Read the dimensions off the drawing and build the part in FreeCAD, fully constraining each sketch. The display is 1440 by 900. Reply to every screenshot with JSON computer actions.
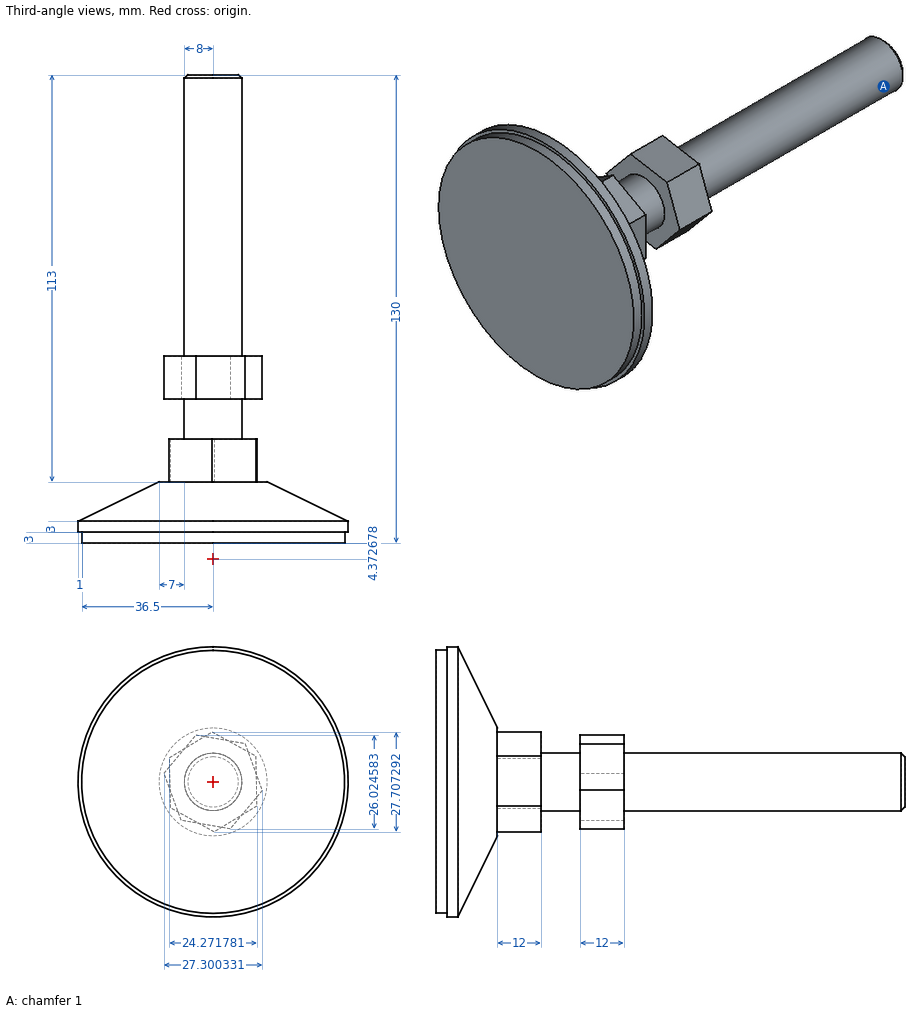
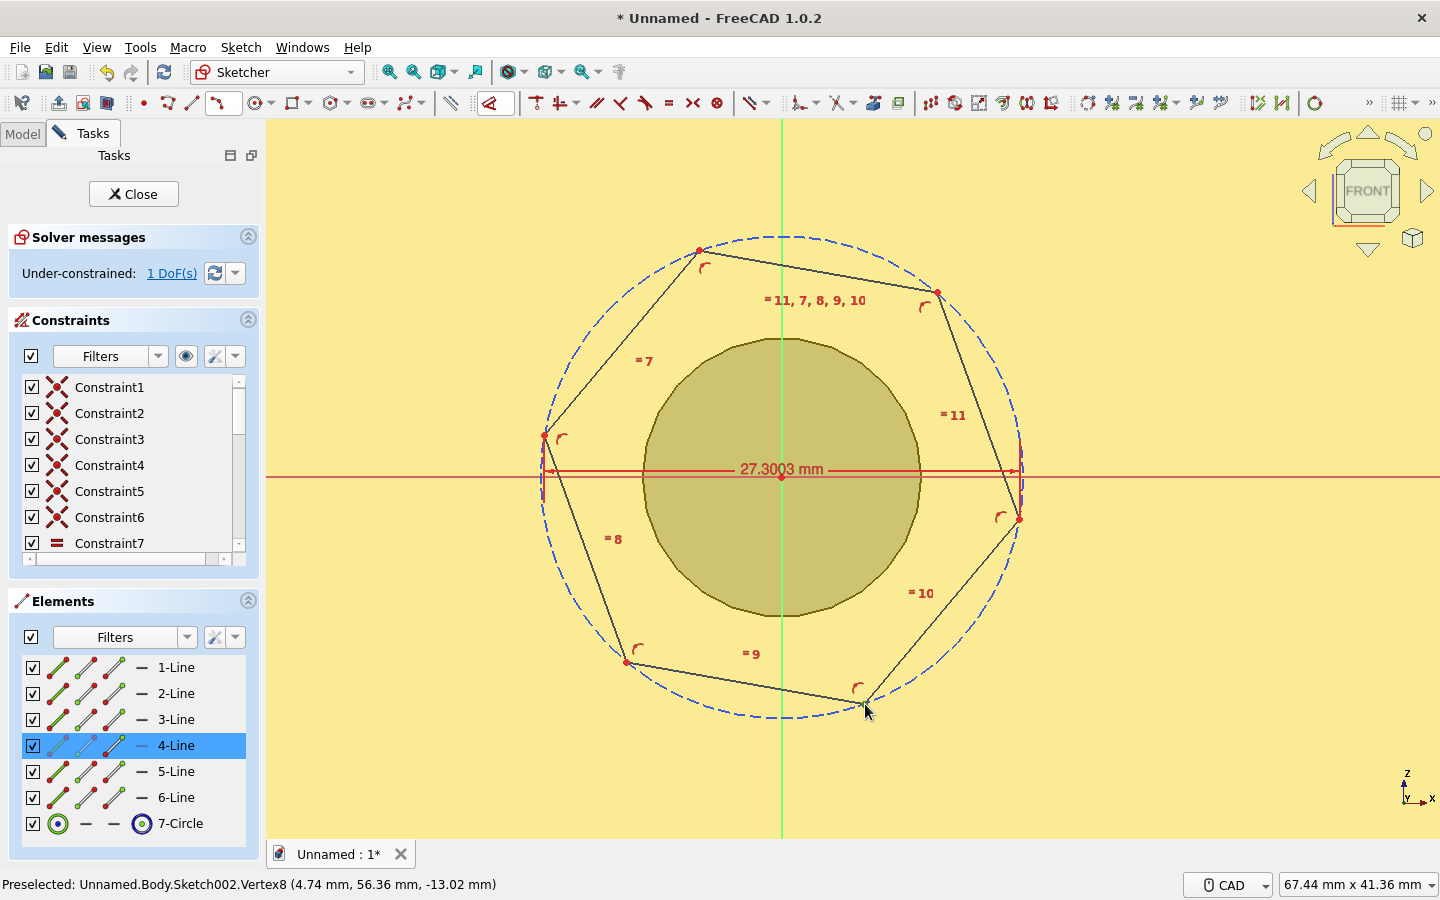
{"action": "left_click", "coordinate": [699, 251]}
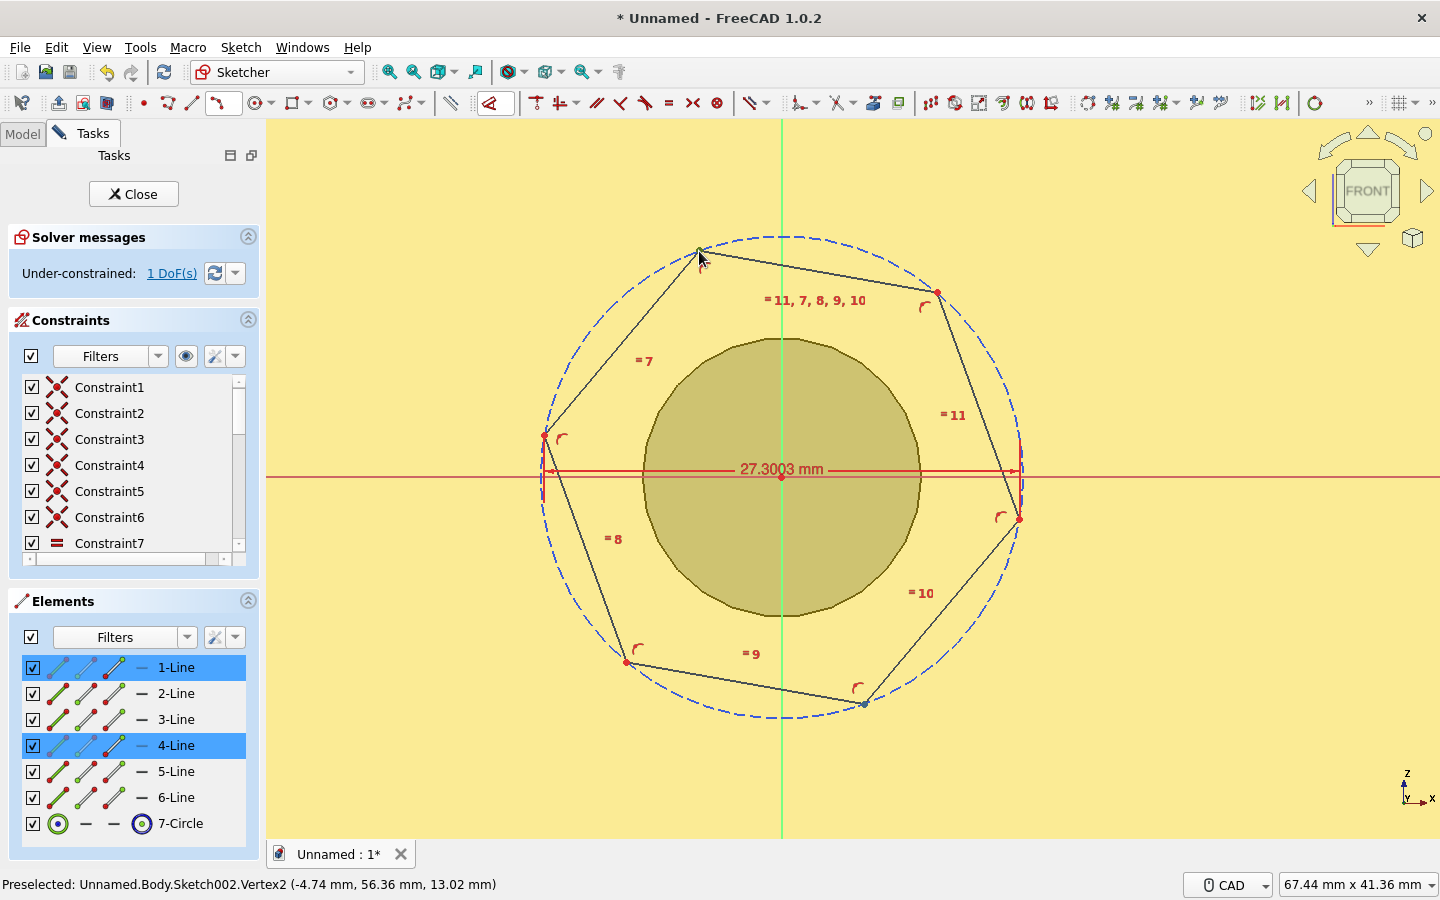
{"action": "left_click", "coordinate": [508, 104]}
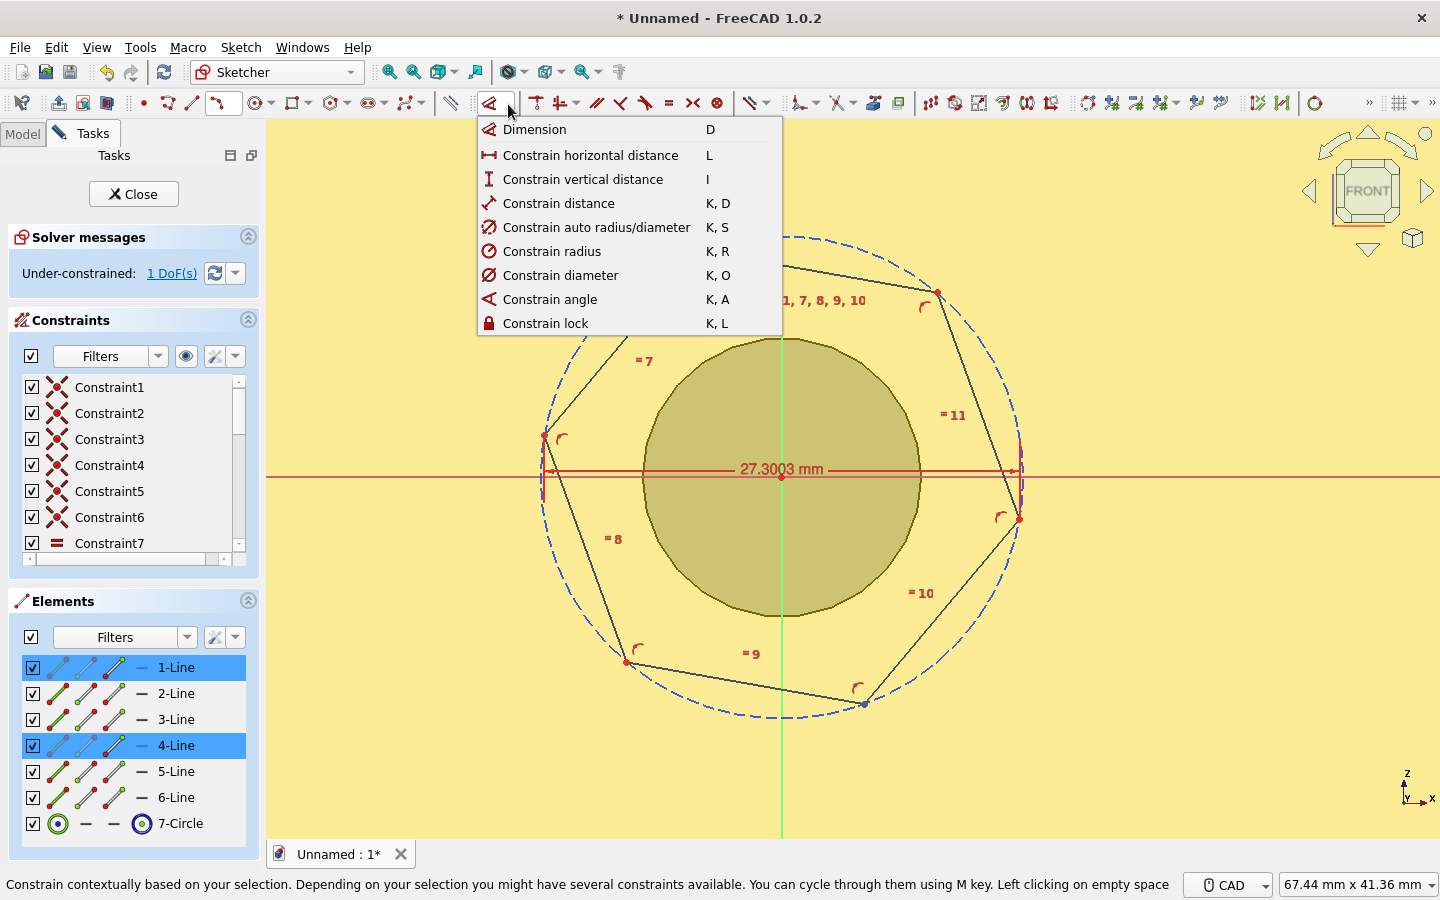
{"action": "left_click", "coordinate": [630, 179]}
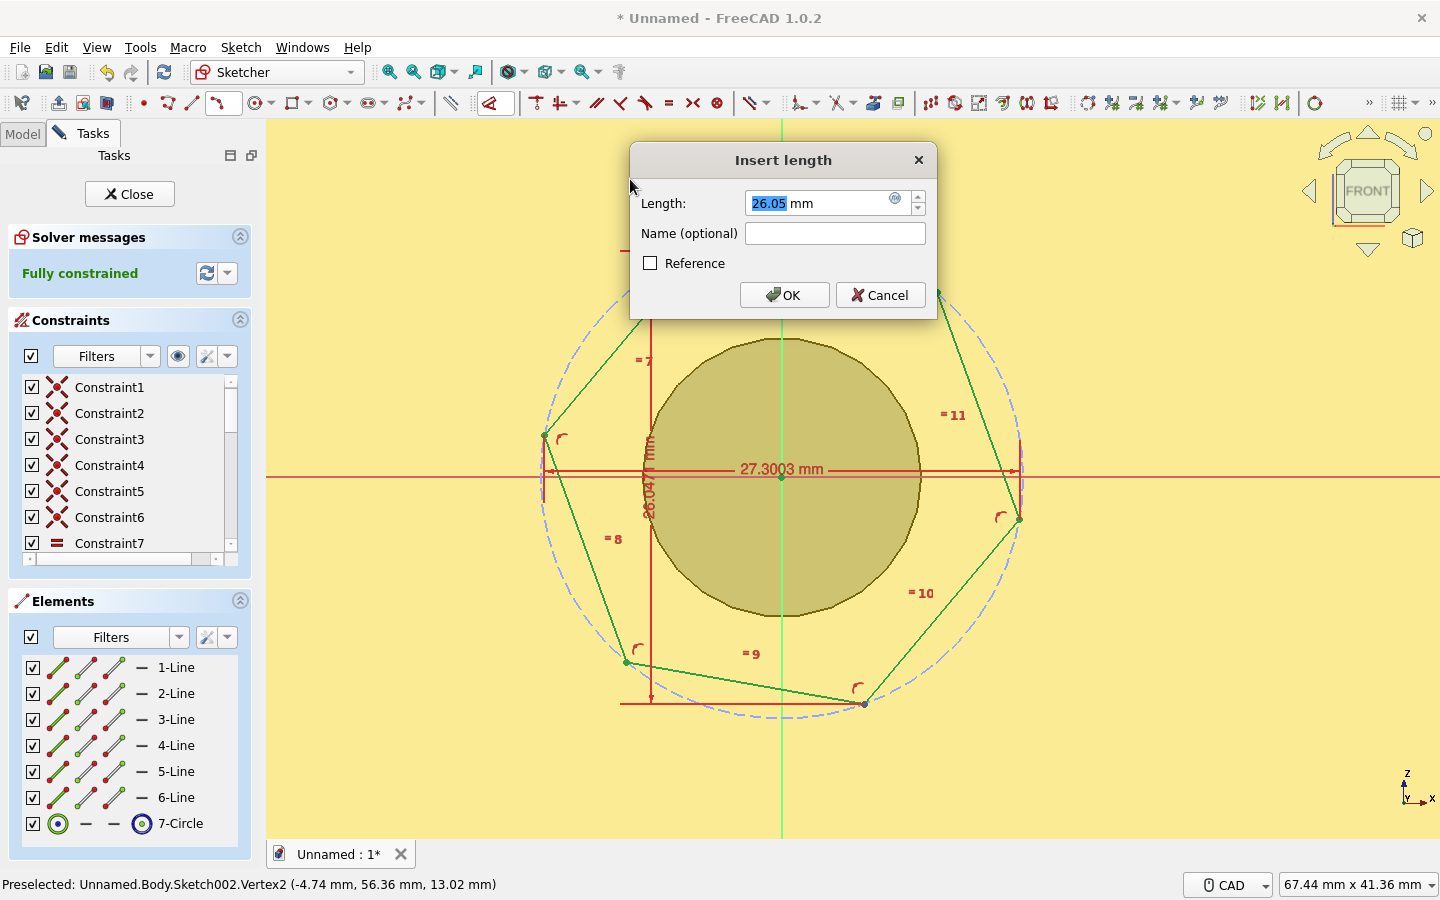
{"action": "type", "text": "26.024583"}
{"action": "key", "text": "Return"}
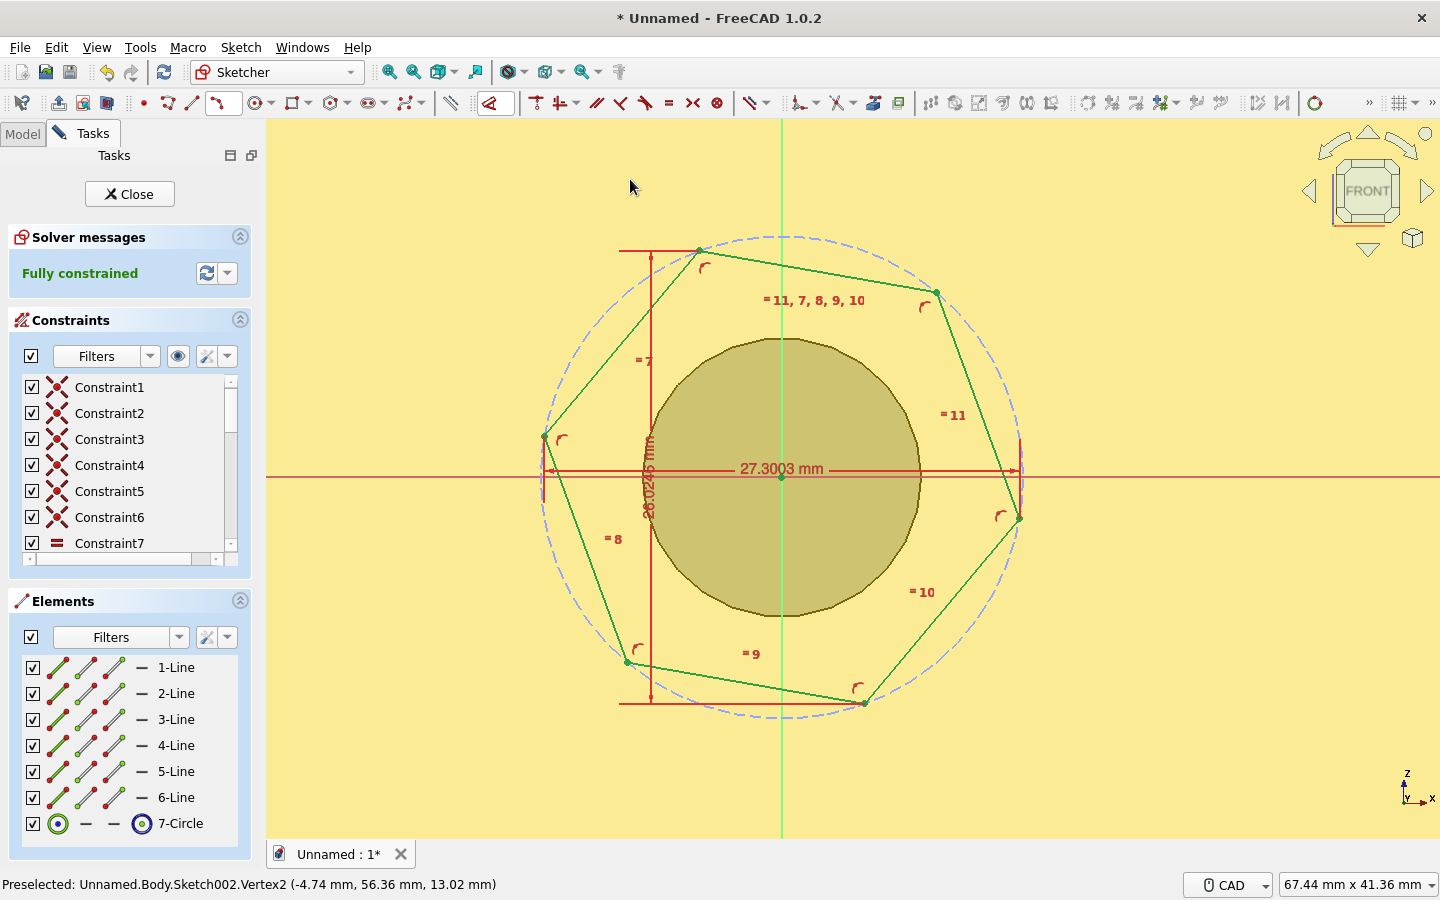
{"action": "left_click", "coordinate": [130, 194]}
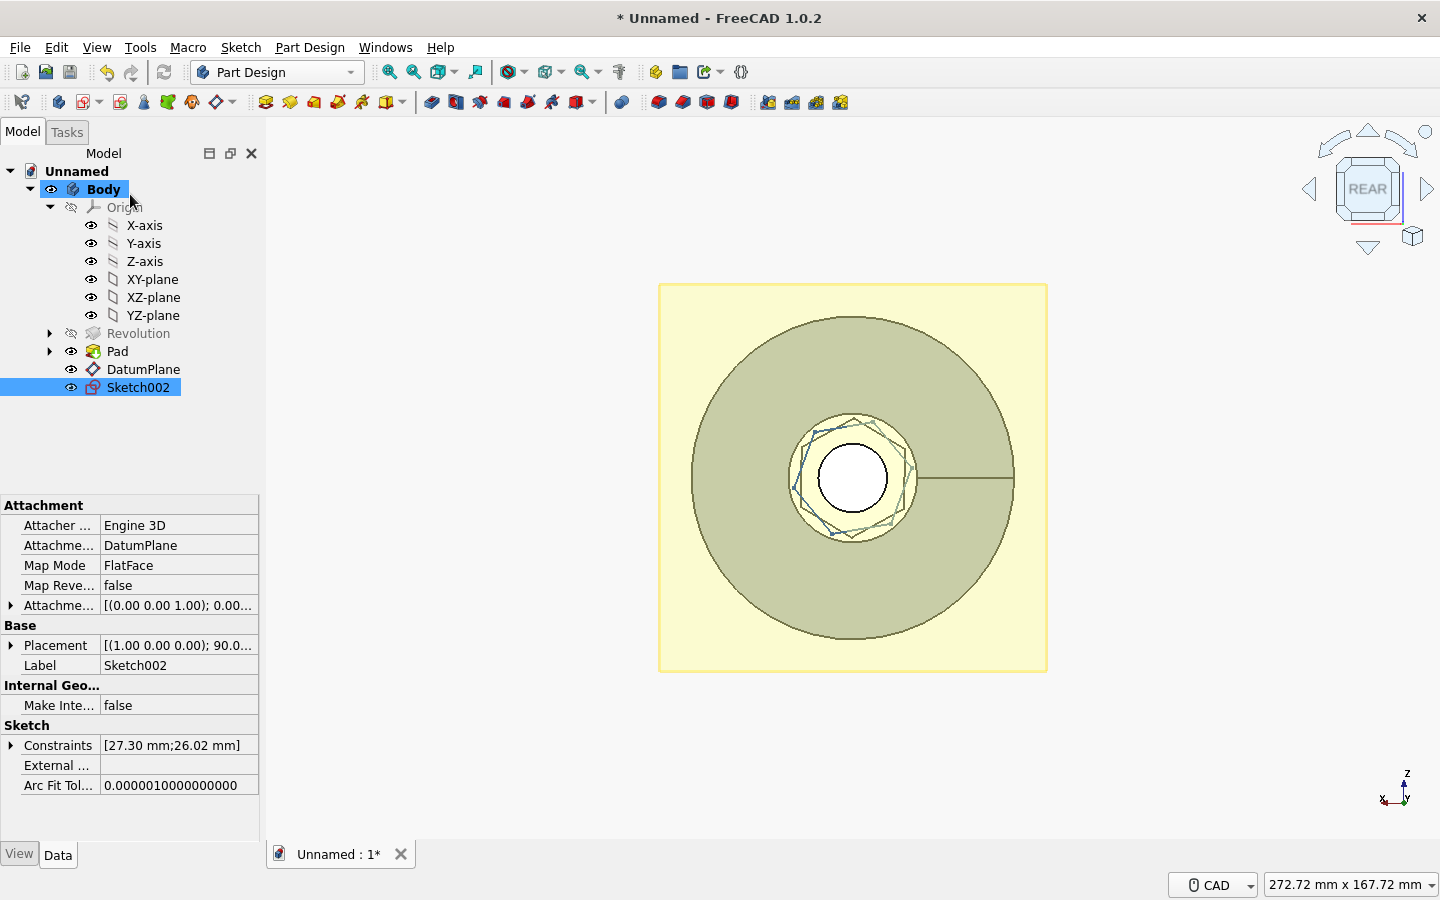
{"action": "left_click", "coordinate": [266, 102]}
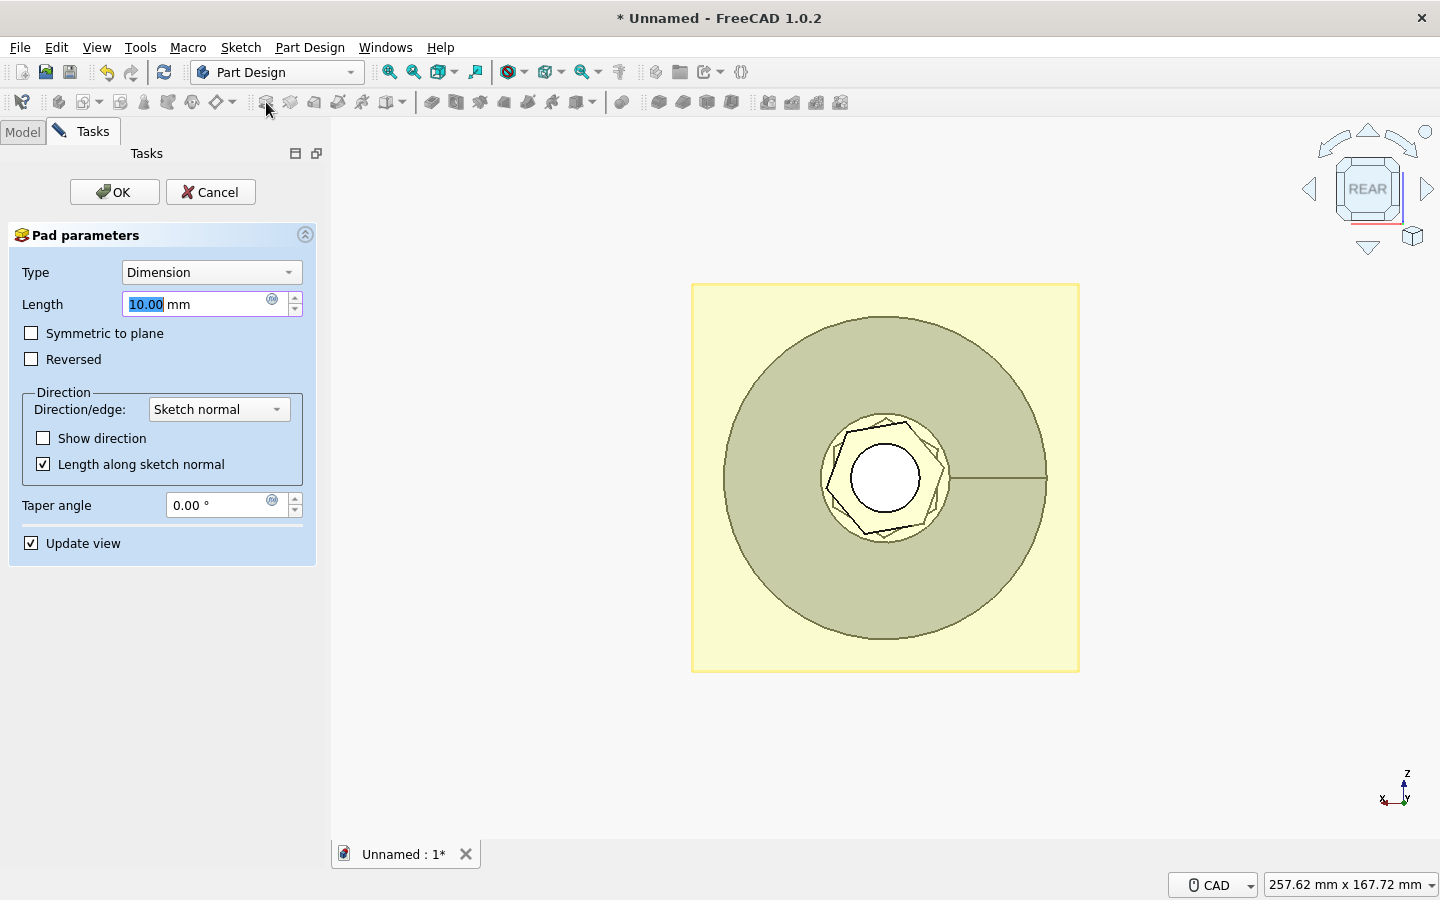
{"action": "type", "text": "12"}
{"action": "key", "text": "Tab"}